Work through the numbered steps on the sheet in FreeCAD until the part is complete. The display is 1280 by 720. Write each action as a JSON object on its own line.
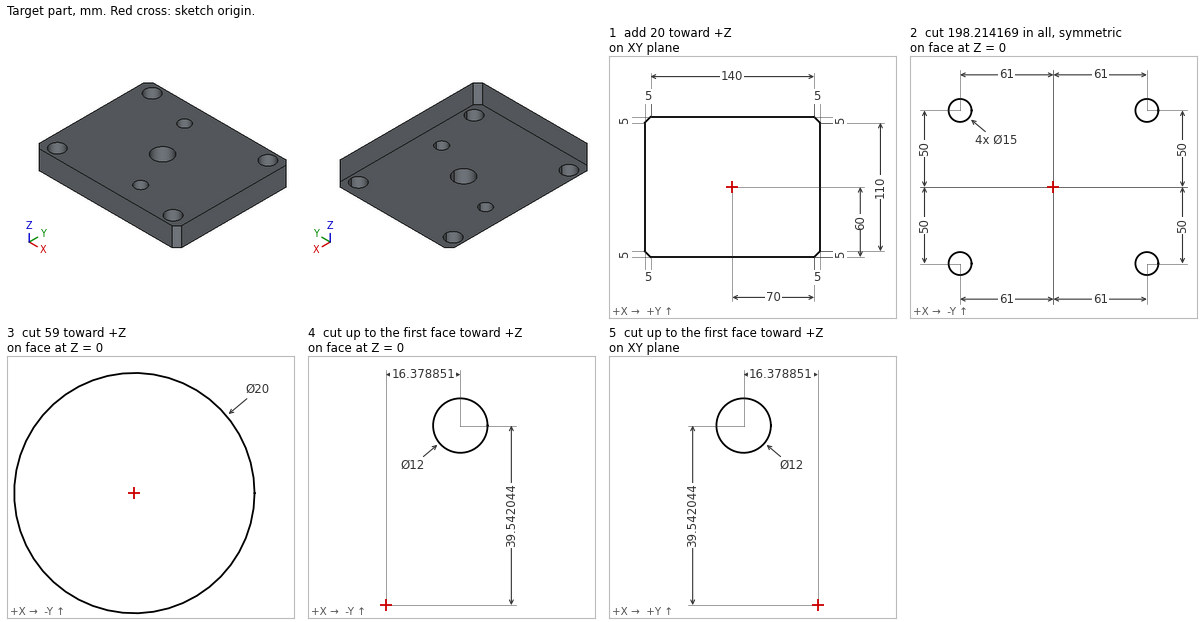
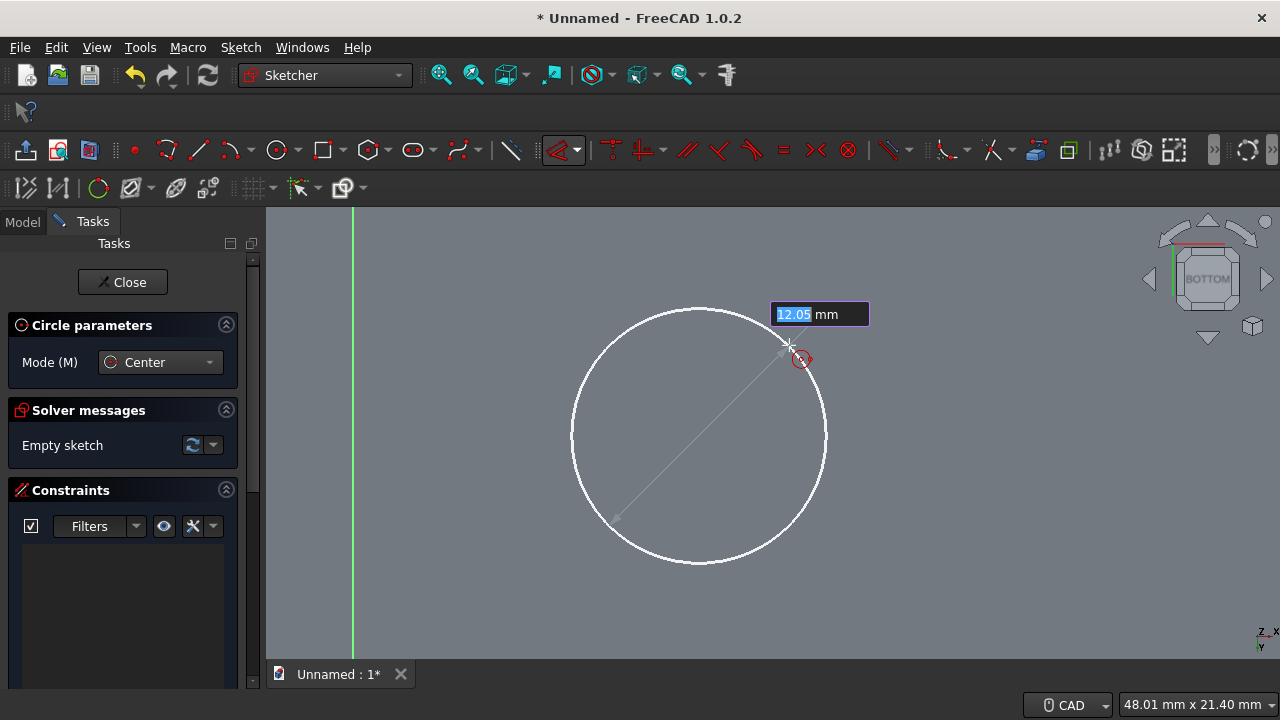
{"action": "type", "text": "12"}
{"action": "key", "text": "Return"}
{"action": "key", "text": "Escape"}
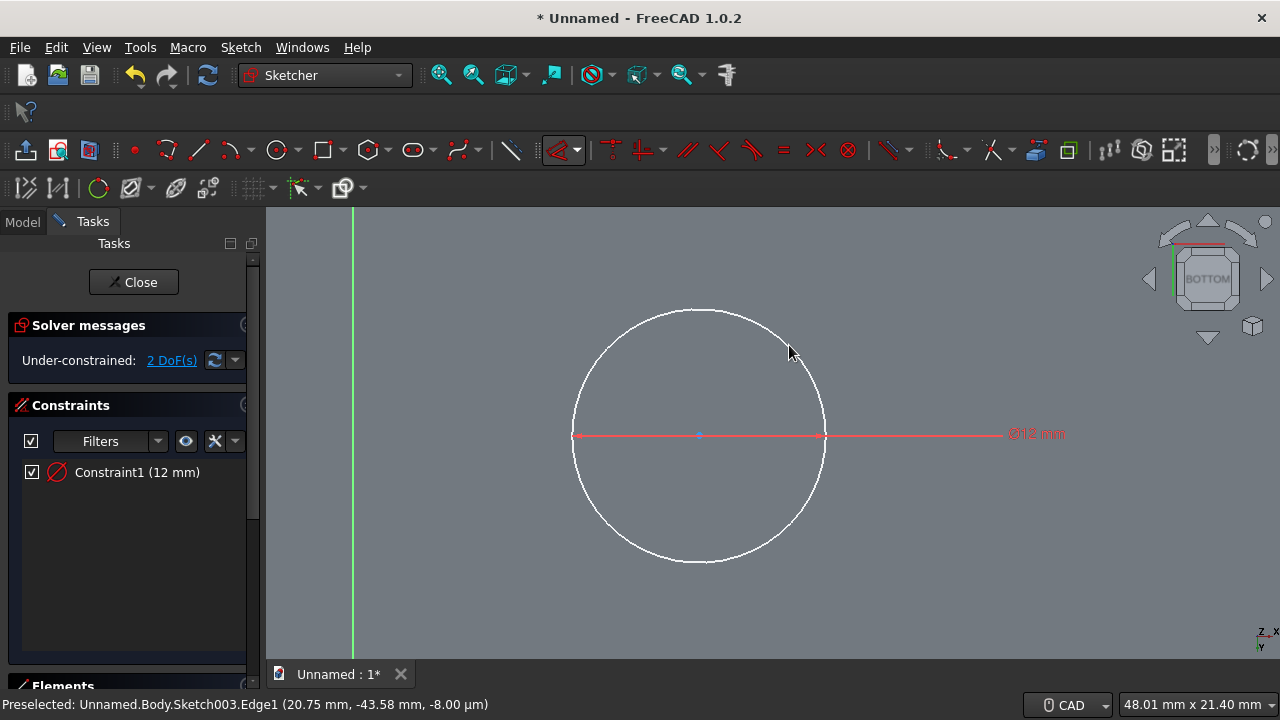
{"action": "left_click", "coordinate": [699, 436]}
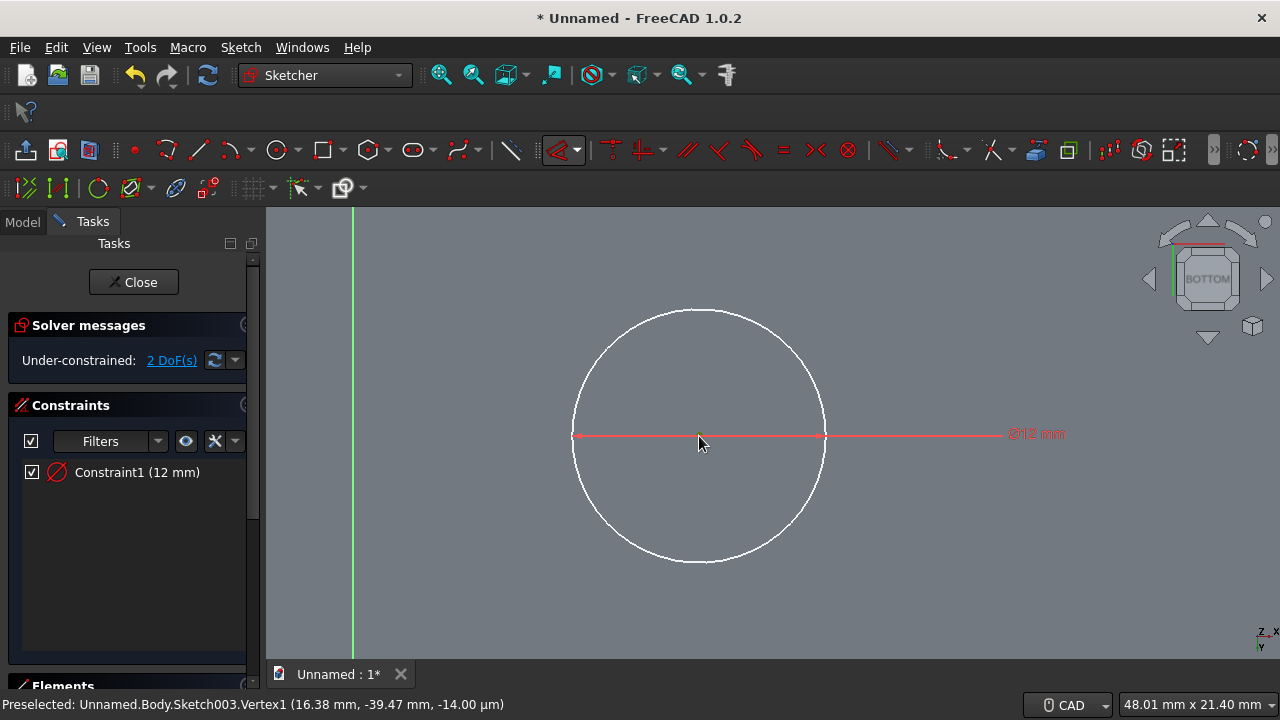
{"action": "key", "text": "l"}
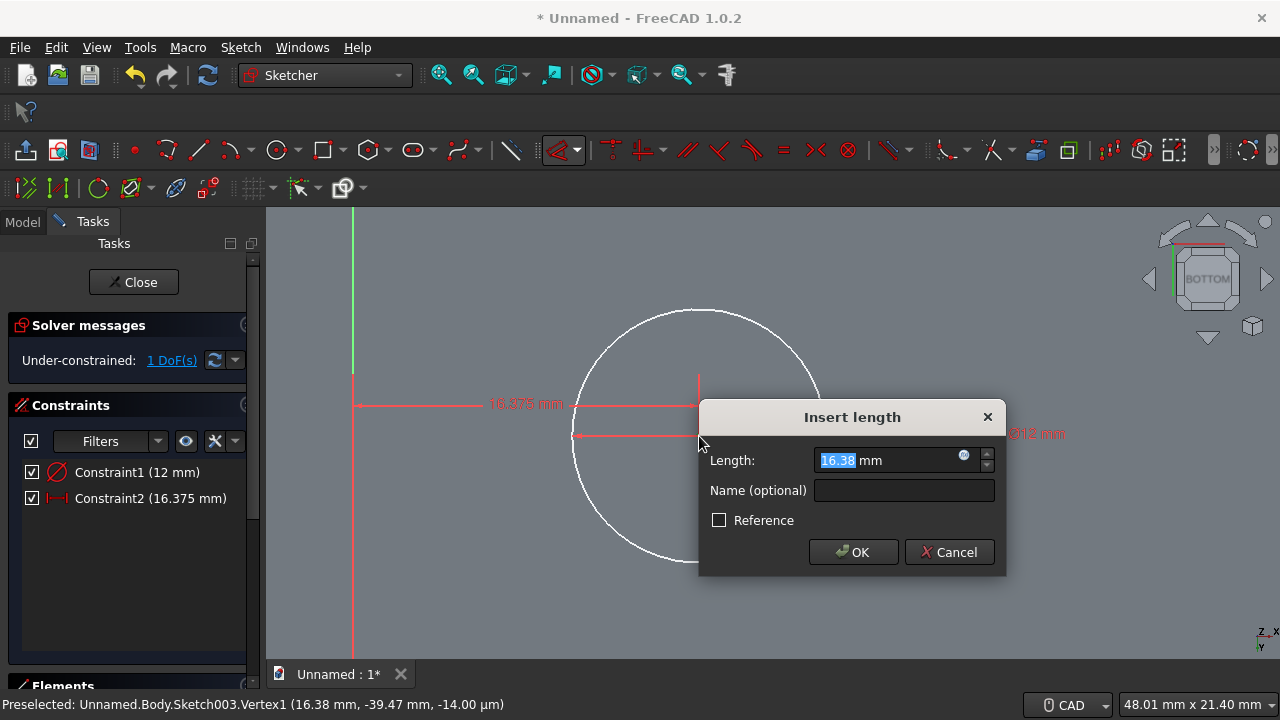
{"action": "type", "text": "16.378851"}
{"action": "key", "text": "Return"}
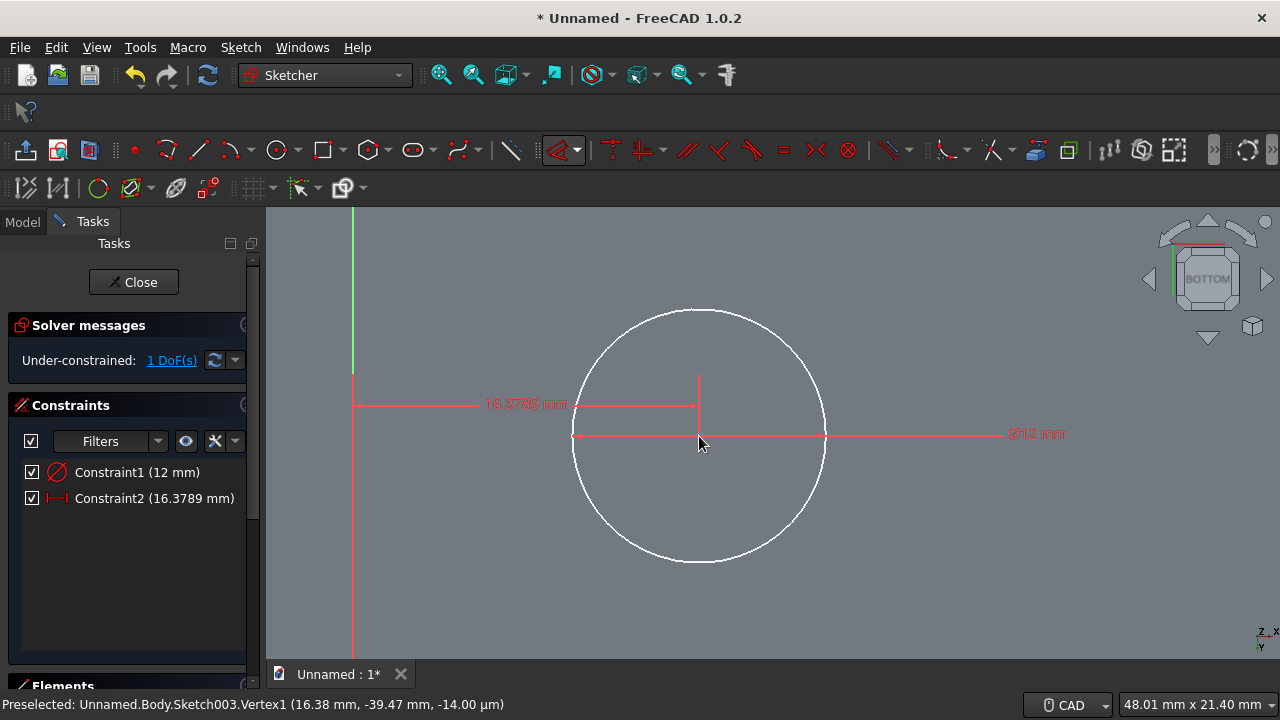
{"action": "left_click", "coordinate": [699, 436]}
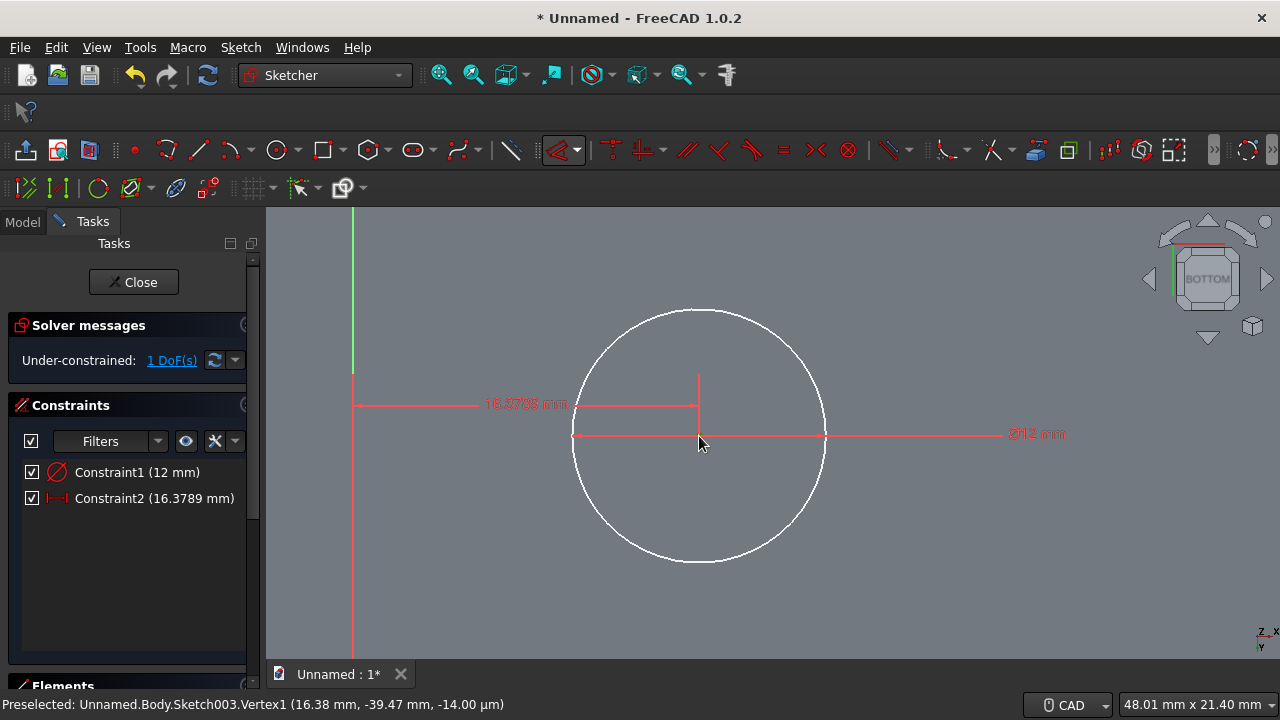
{"action": "key", "text": "i"}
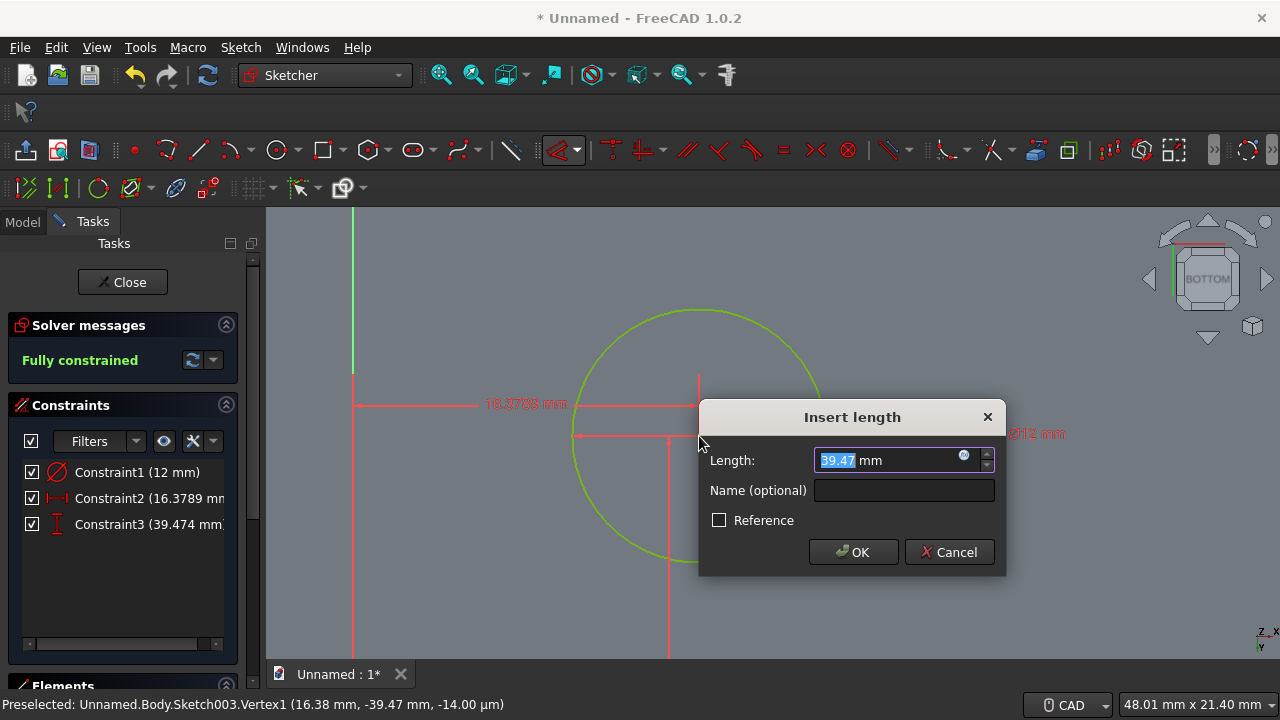
{"action": "type", "text": "39.542044"}
{"action": "key", "text": "Return"}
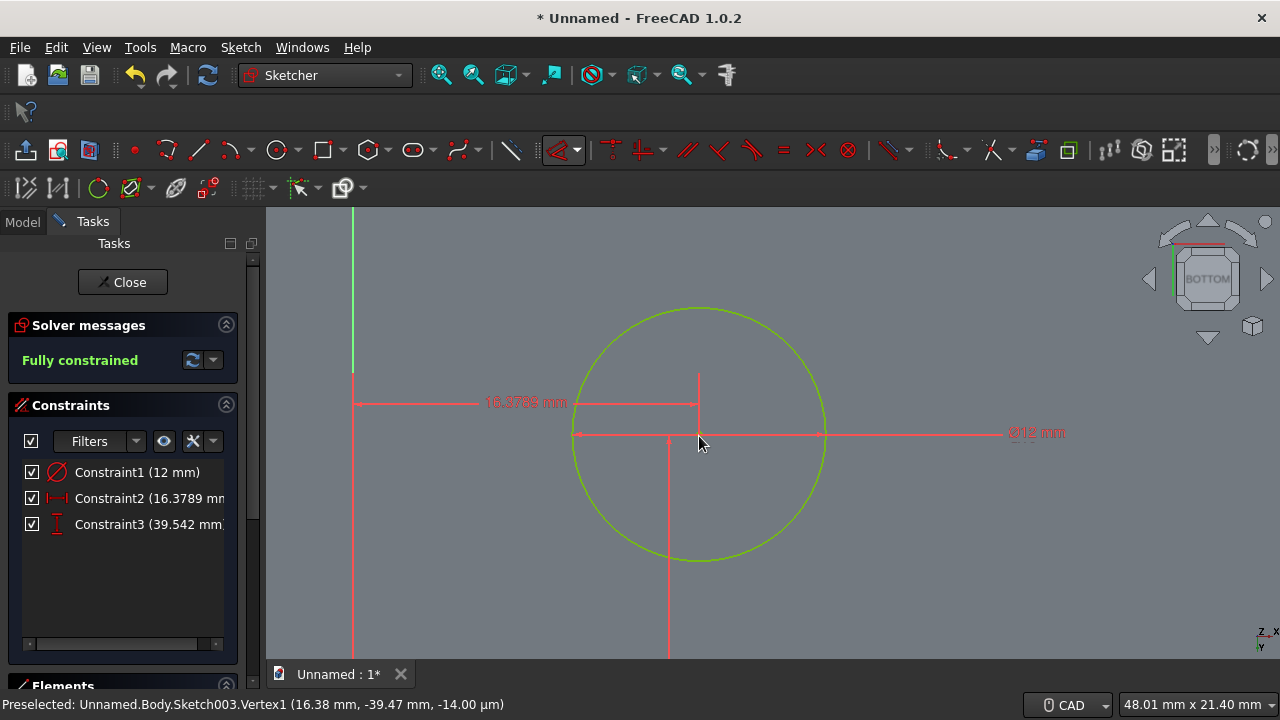
{"action": "left_click", "coordinate": [123, 282]}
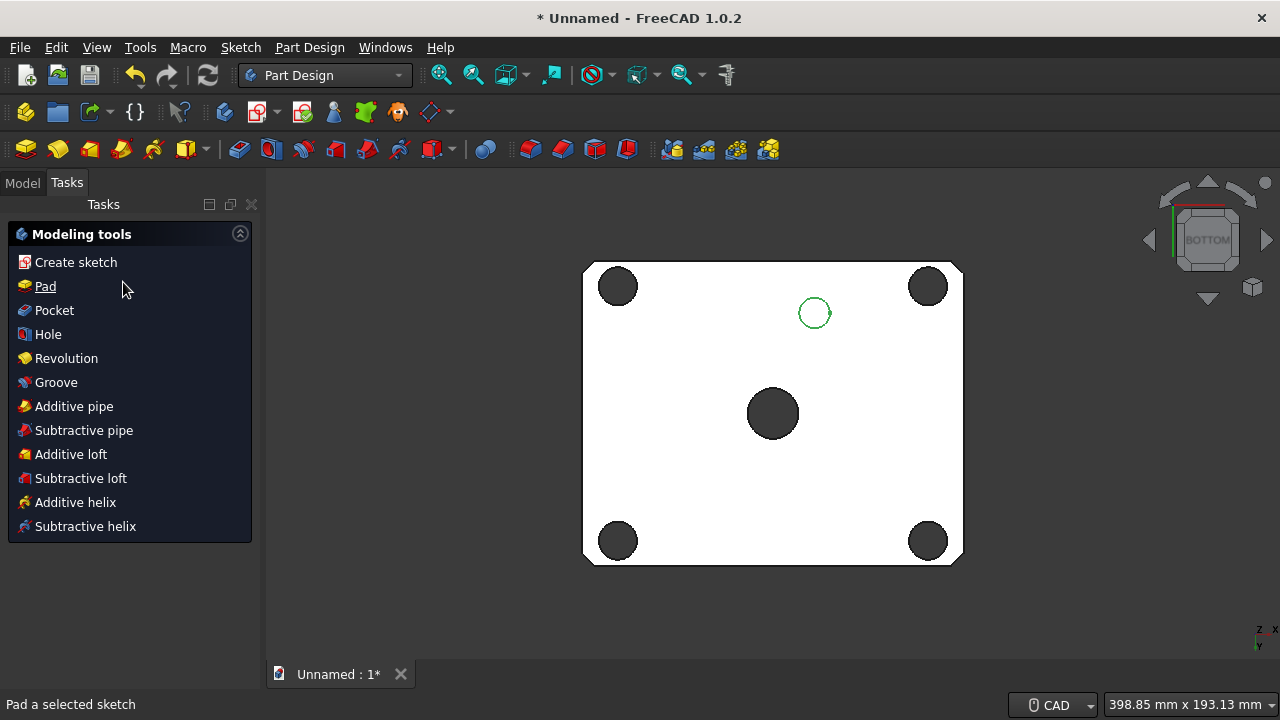
{"action": "left_click", "coordinate": [240, 150]}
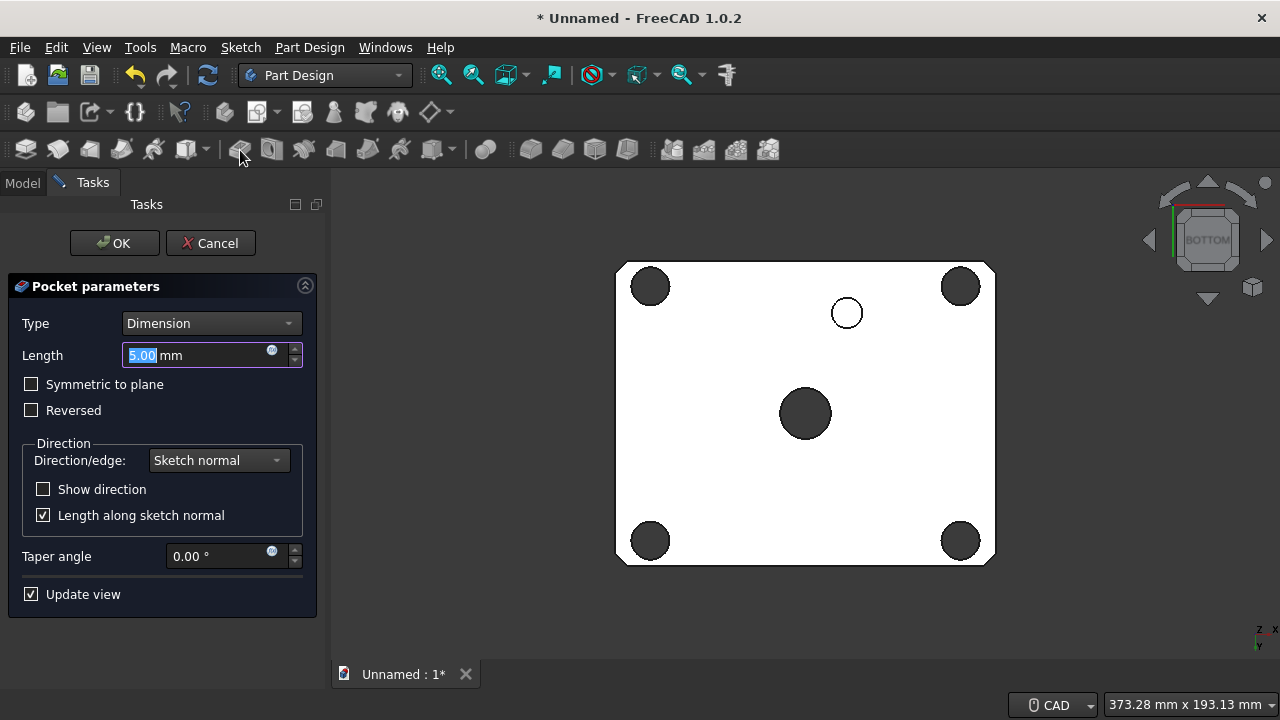
{"action": "left_click", "coordinate": [212, 324]}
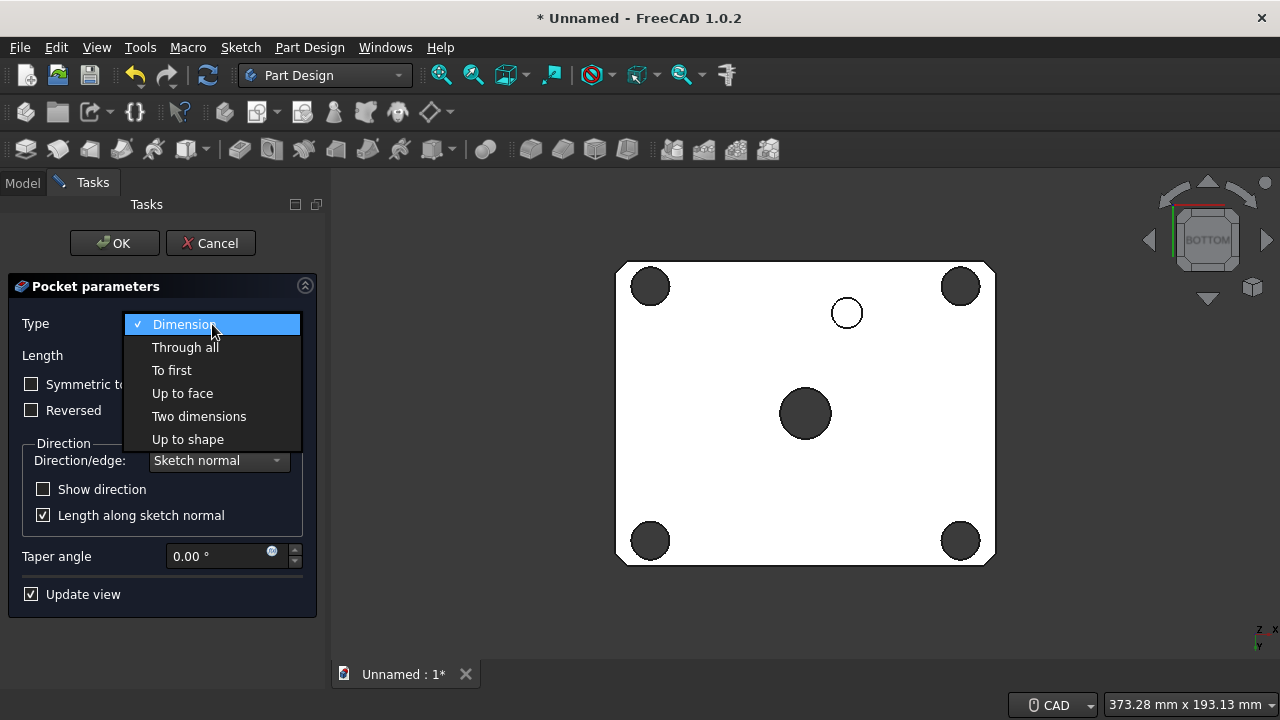
{"action": "left_click", "coordinate": [212, 370]}